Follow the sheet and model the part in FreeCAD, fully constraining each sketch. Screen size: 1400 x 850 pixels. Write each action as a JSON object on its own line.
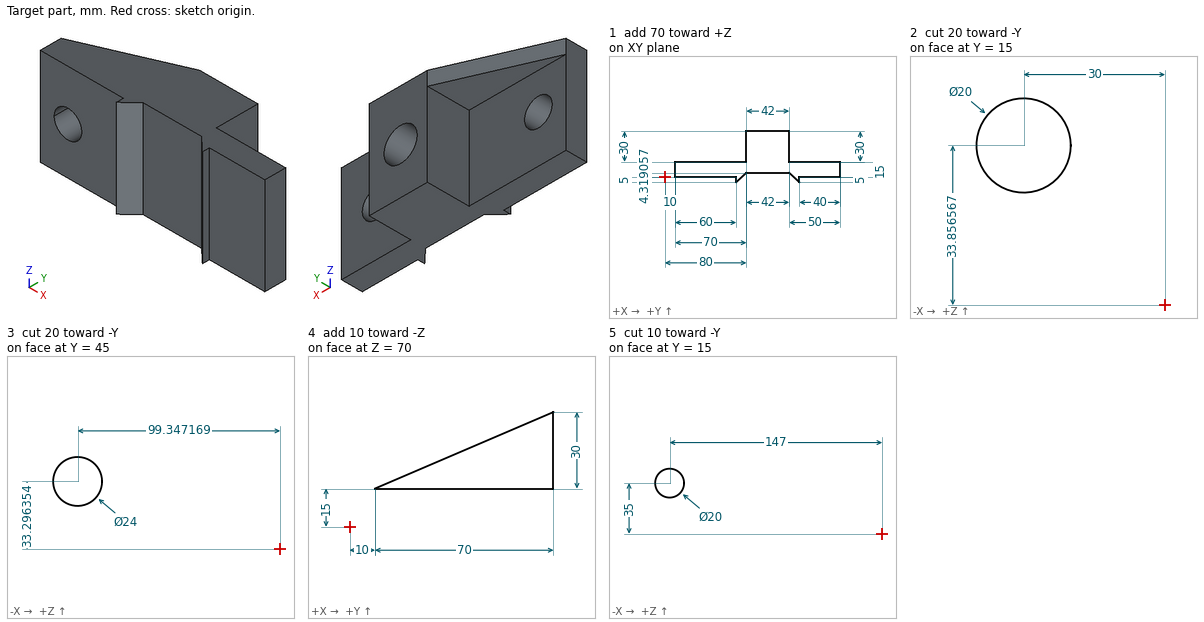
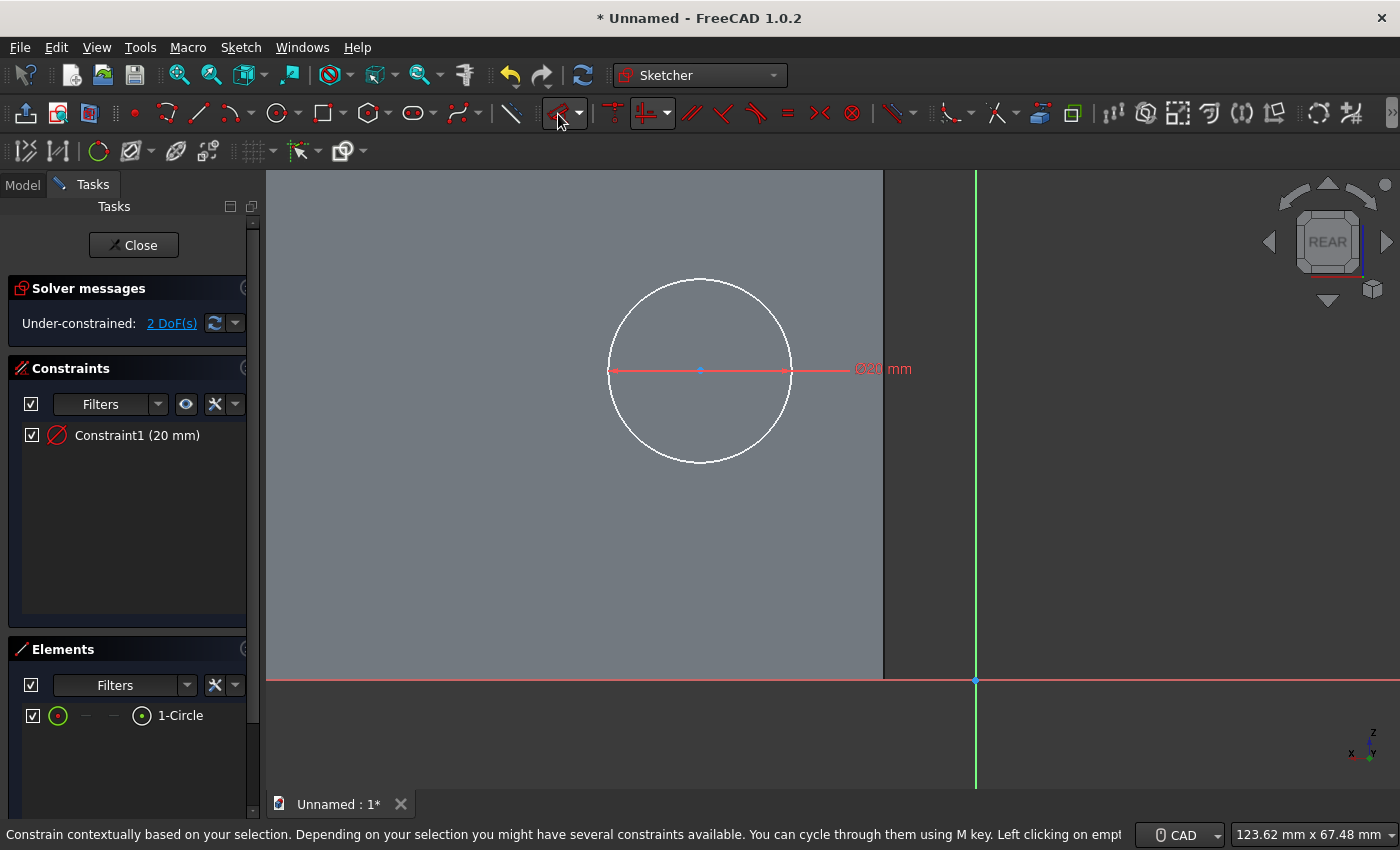
{"action": "left_click", "coordinate": [700, 371]}
{"action": "left_click", "coordinate": [838, 714]}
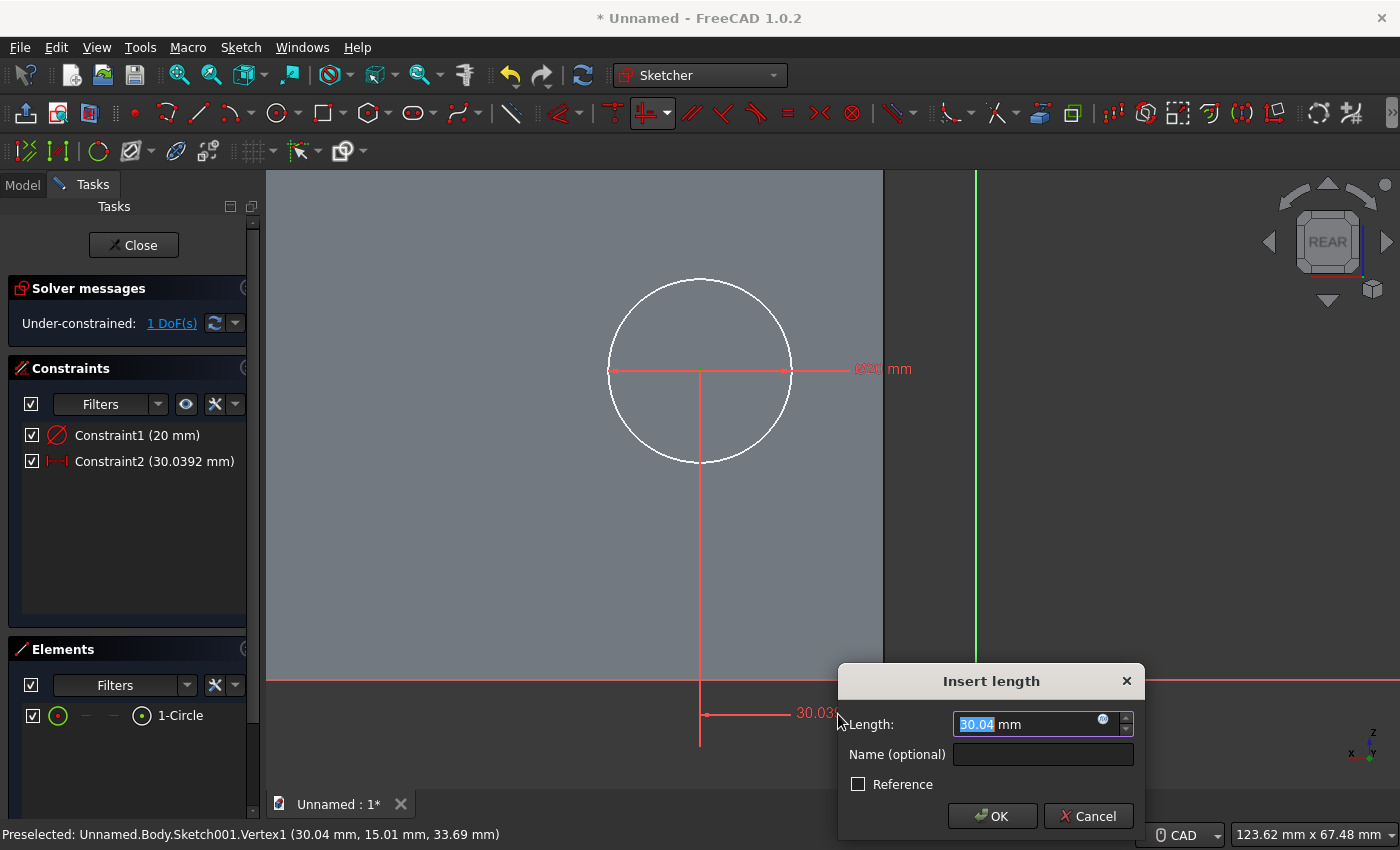
{"action": "type", "text": "30"}
{"action": "key", "text": "Return"}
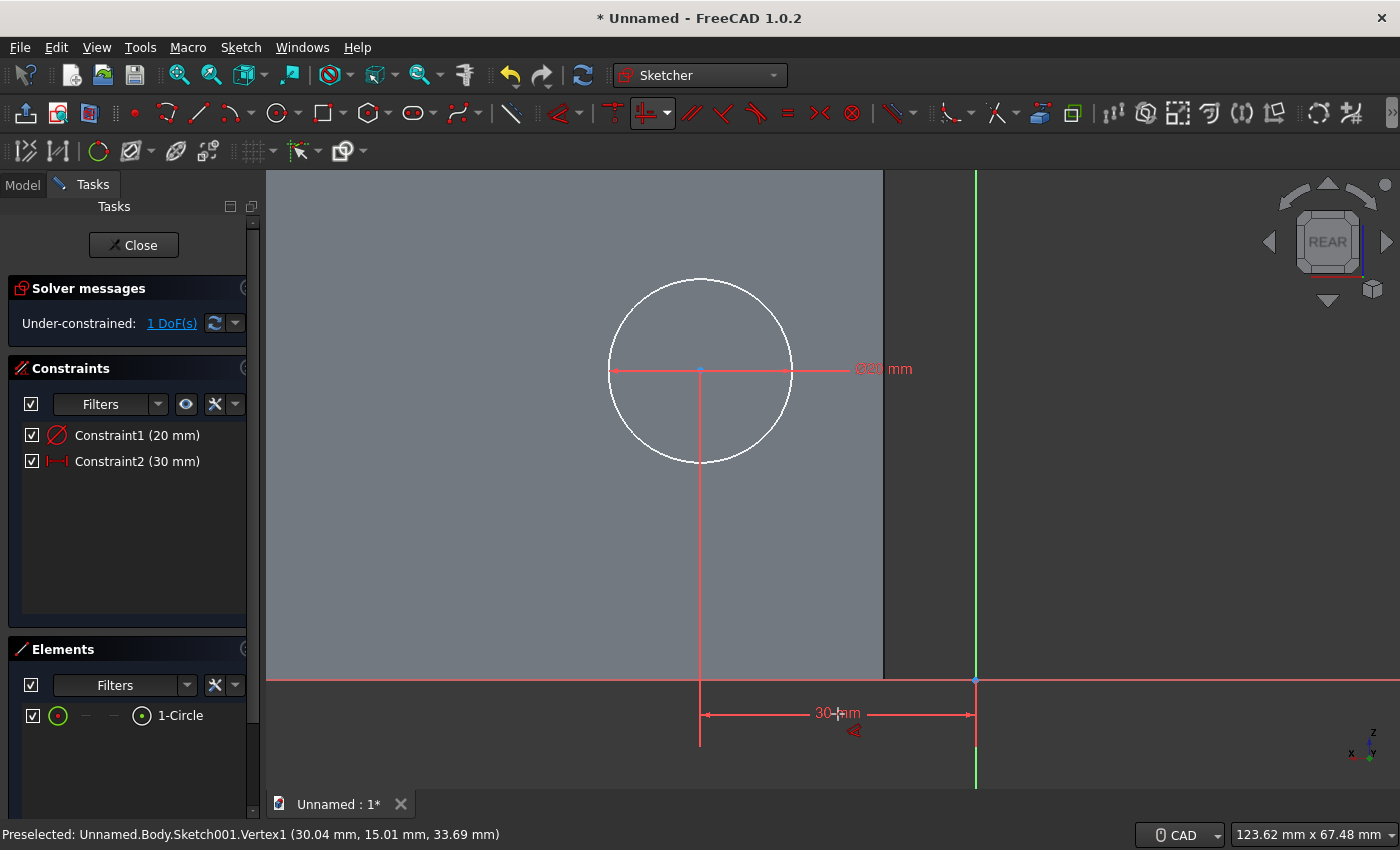
{"action": "left_click", "coordinate": [700, 371]}
{"action": "left_click", "coordinate": [1010, 526]}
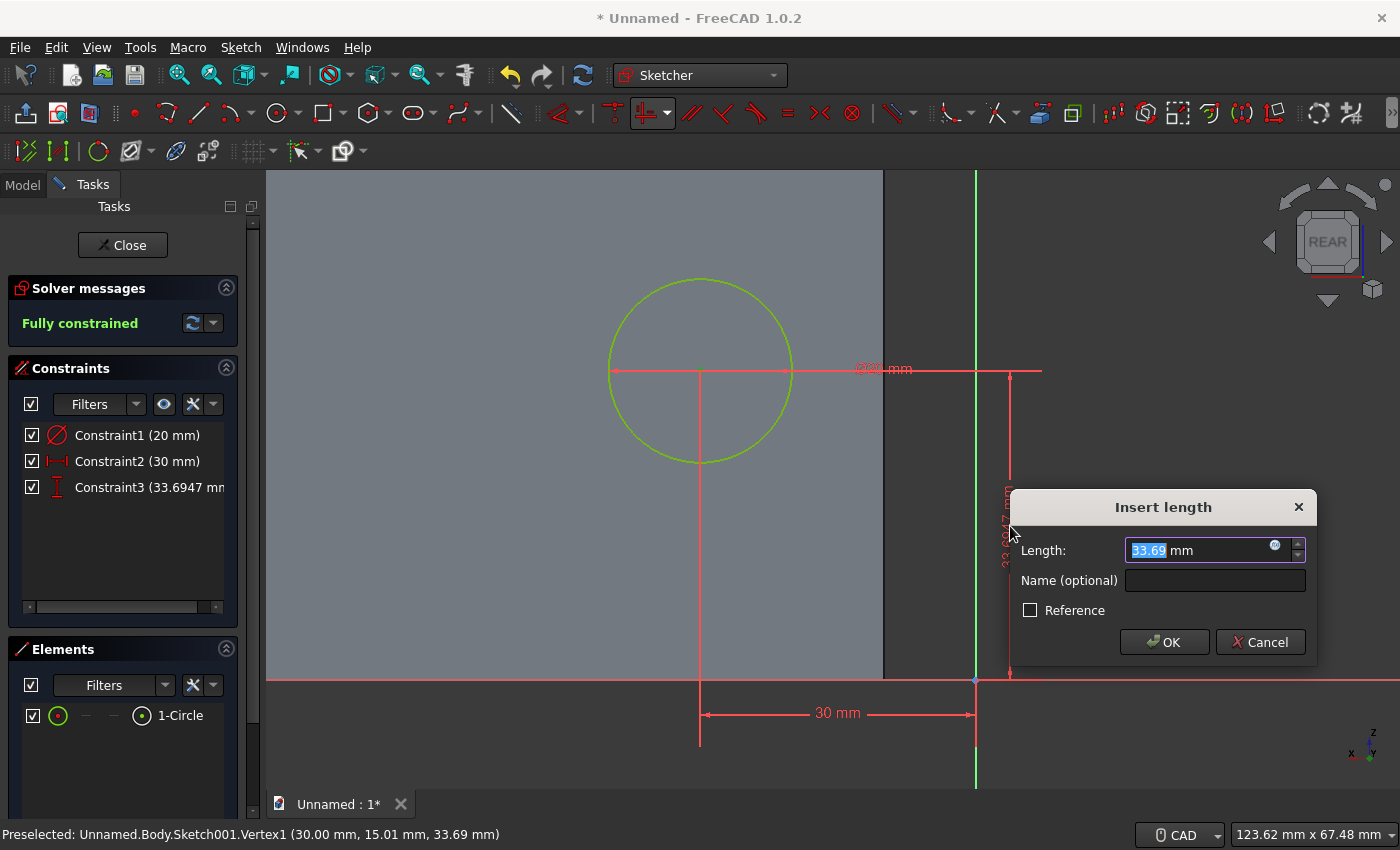
{"action": "type", "text": "33.856567"}
{"action": "key", "text": "Return"}
{"action": "key", "text": "Escape"}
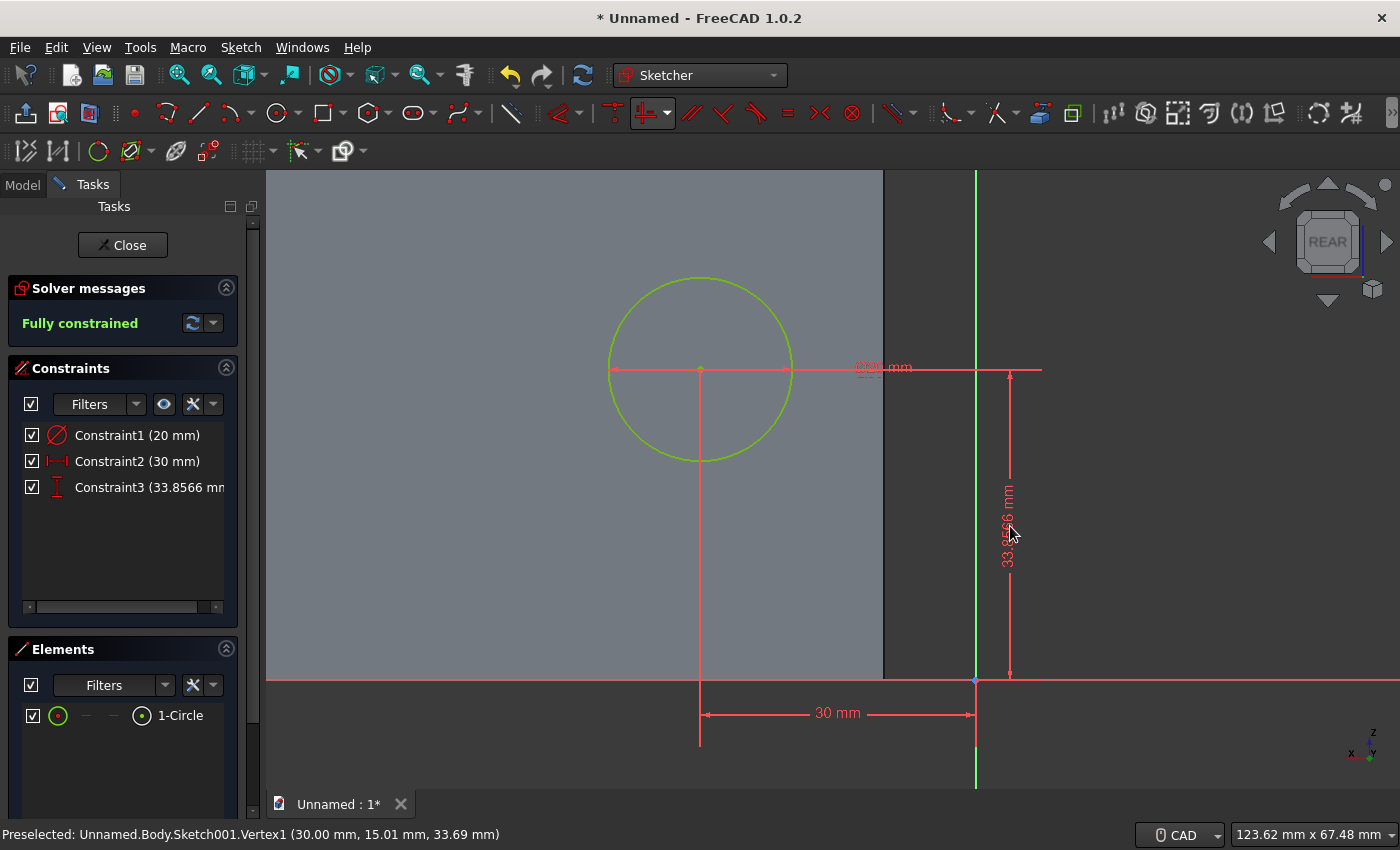
{"action": "left_click", "coordinate": [123, 245]}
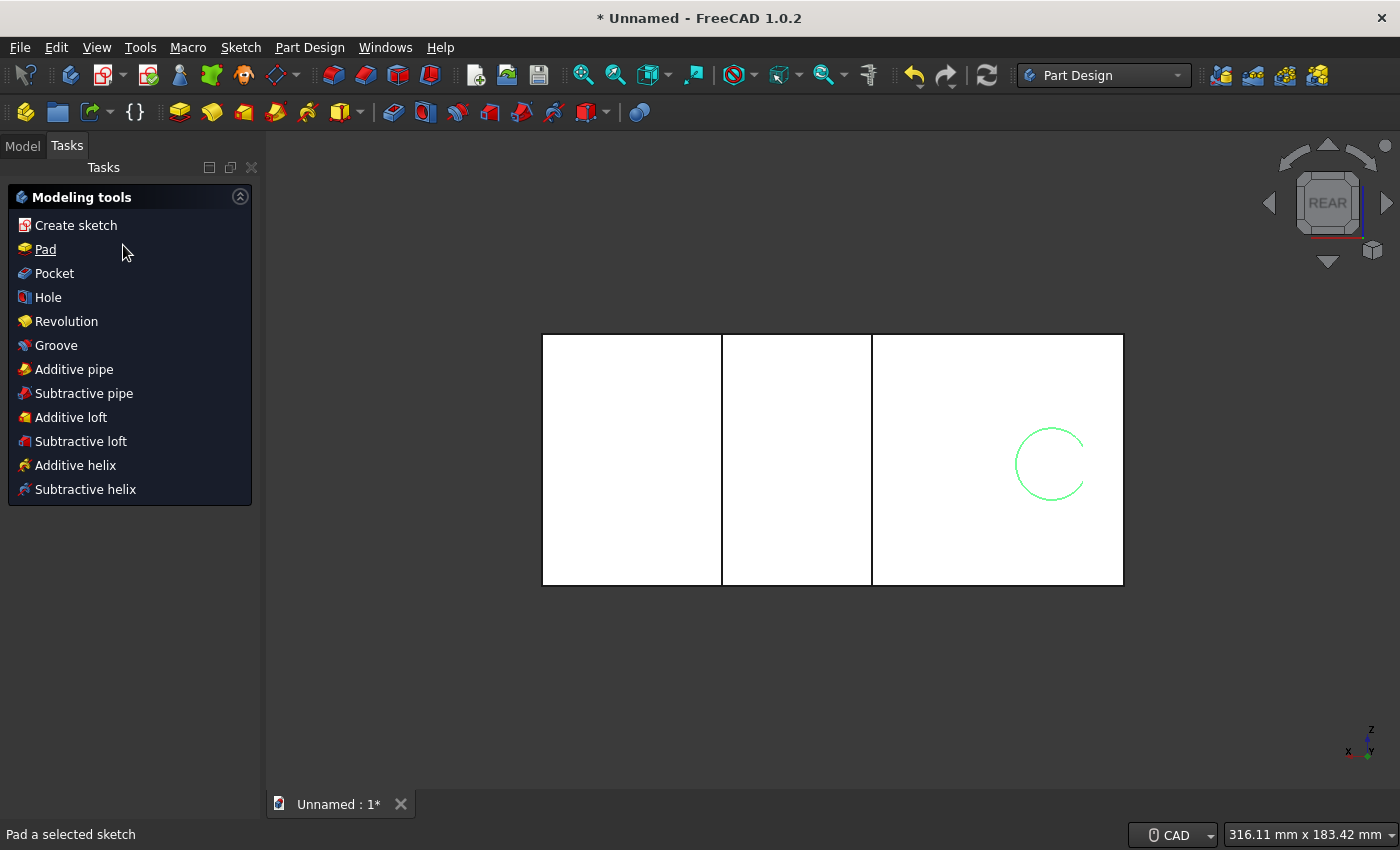
{"action": "left_click", "coordinate": [394, 112]}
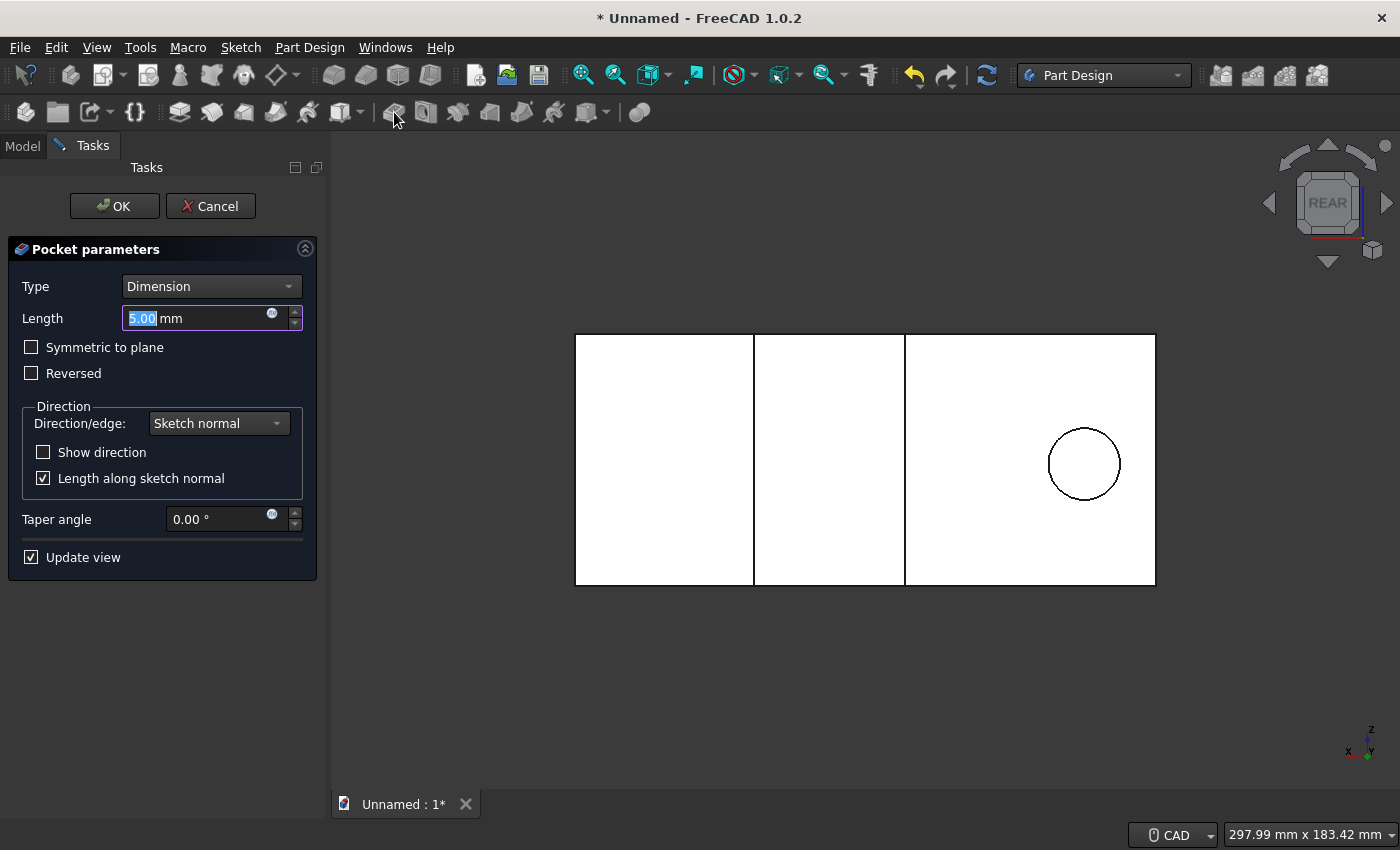
{"action": "type", "text": "20"}
{"action": "key", "text": "Tab"}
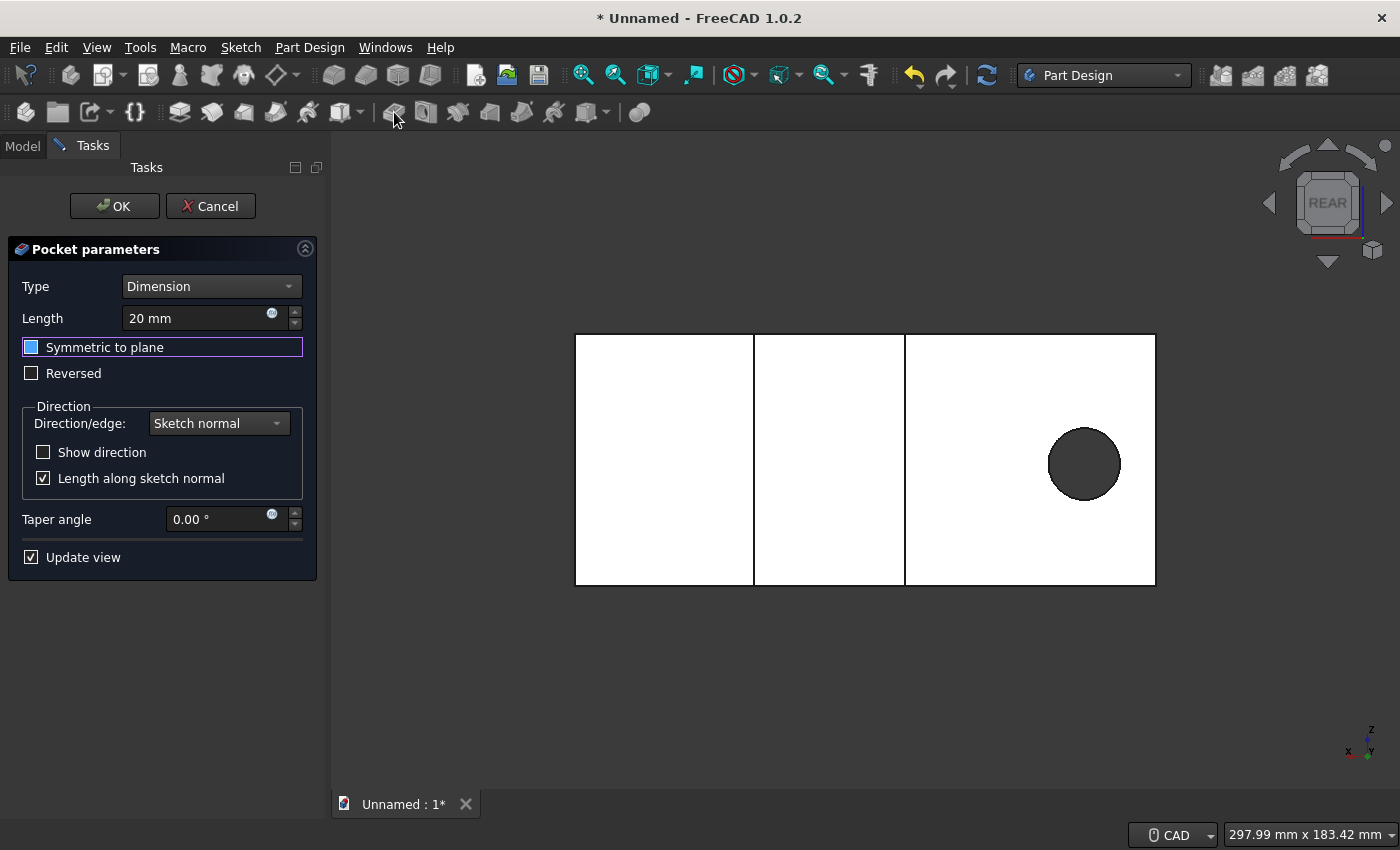
{"action": "left_click", "coordinate": [115, 206]}